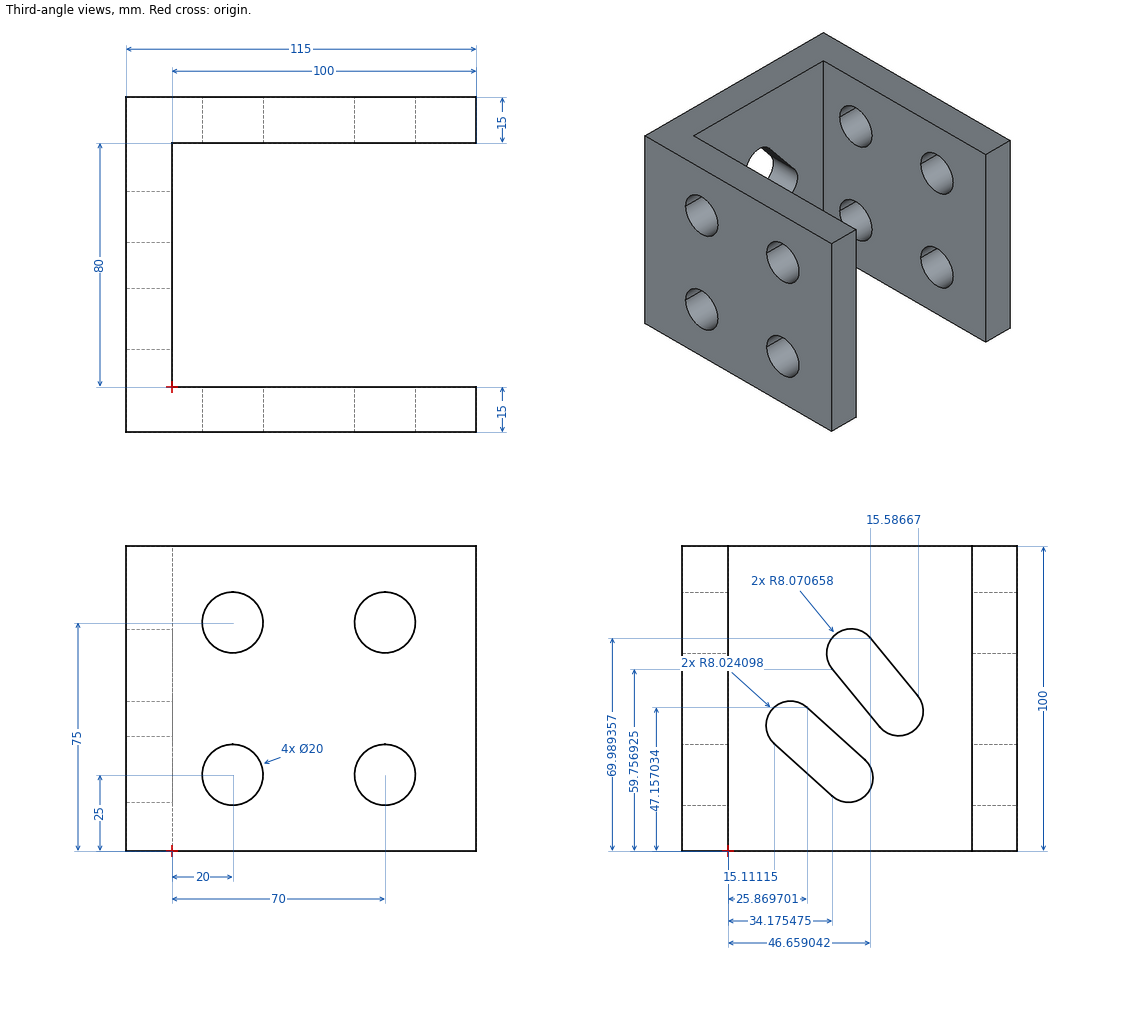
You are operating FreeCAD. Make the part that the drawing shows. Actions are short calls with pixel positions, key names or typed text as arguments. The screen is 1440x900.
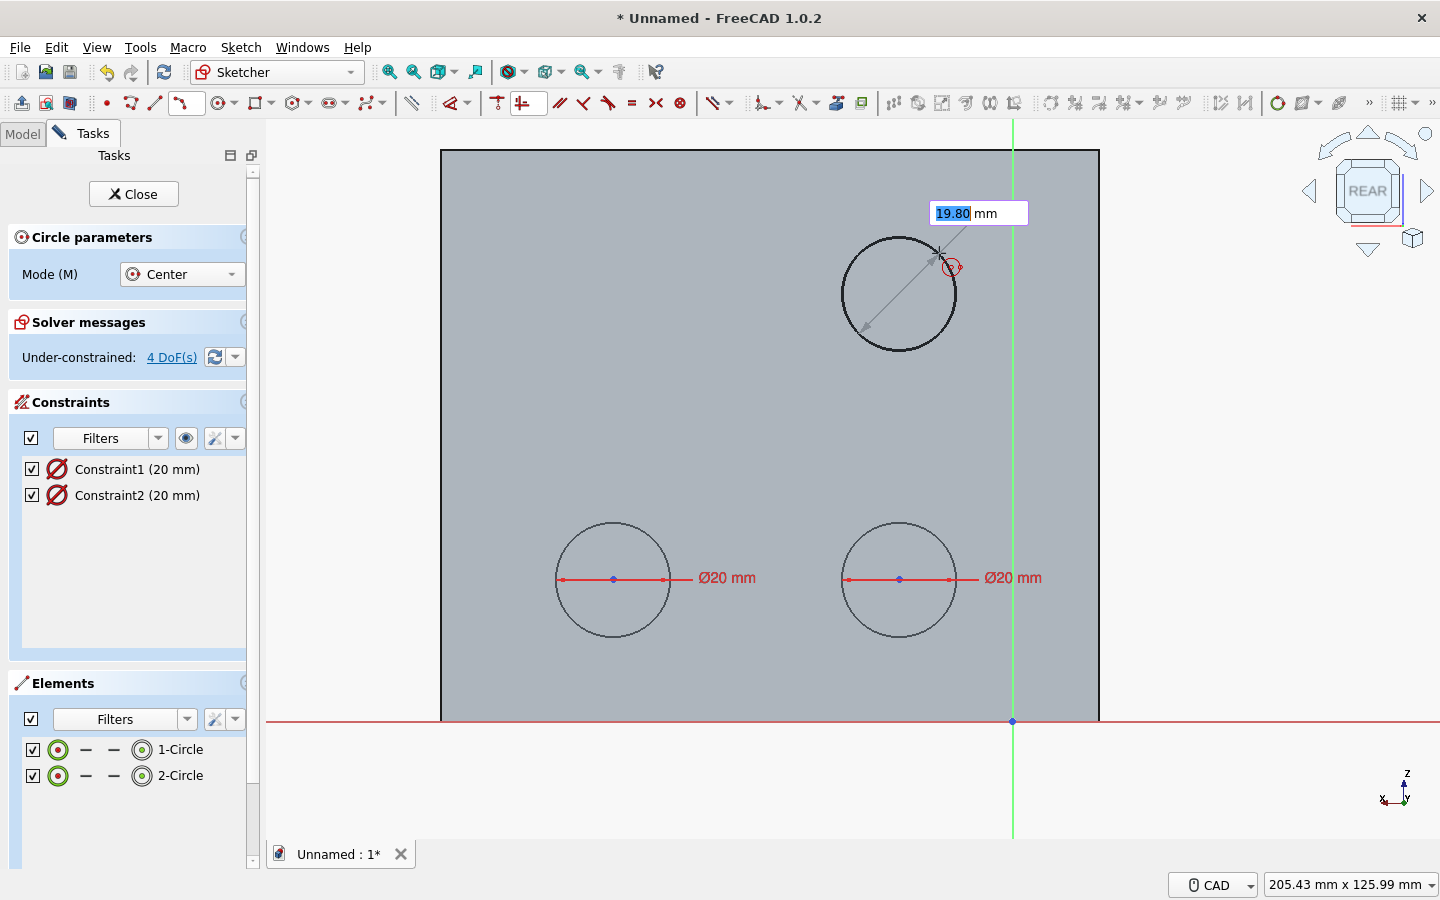
text(20)
key(Return)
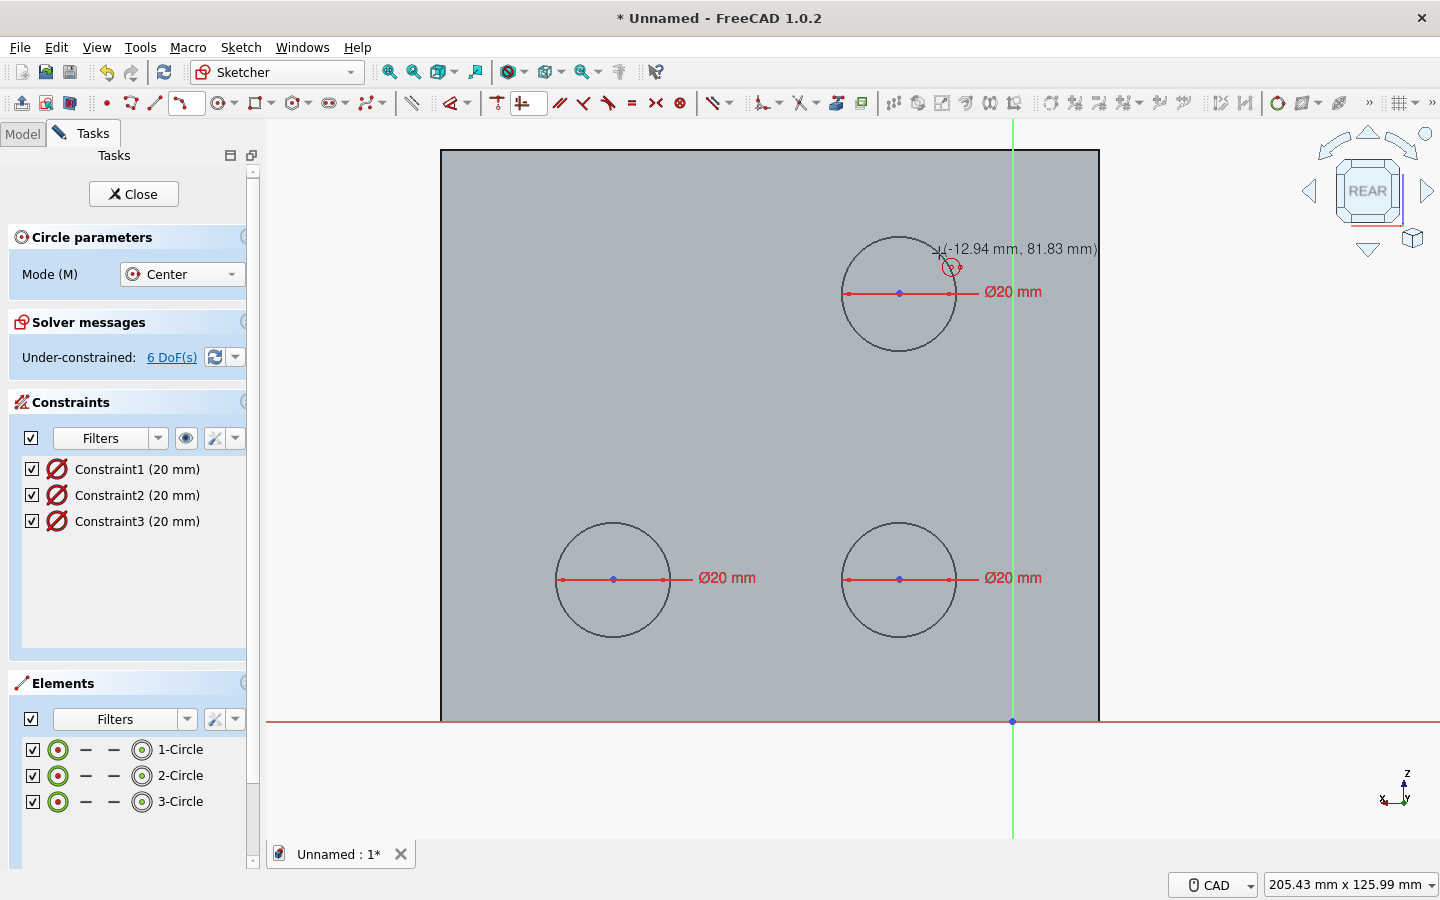
click(613, 293)
move(653, 253)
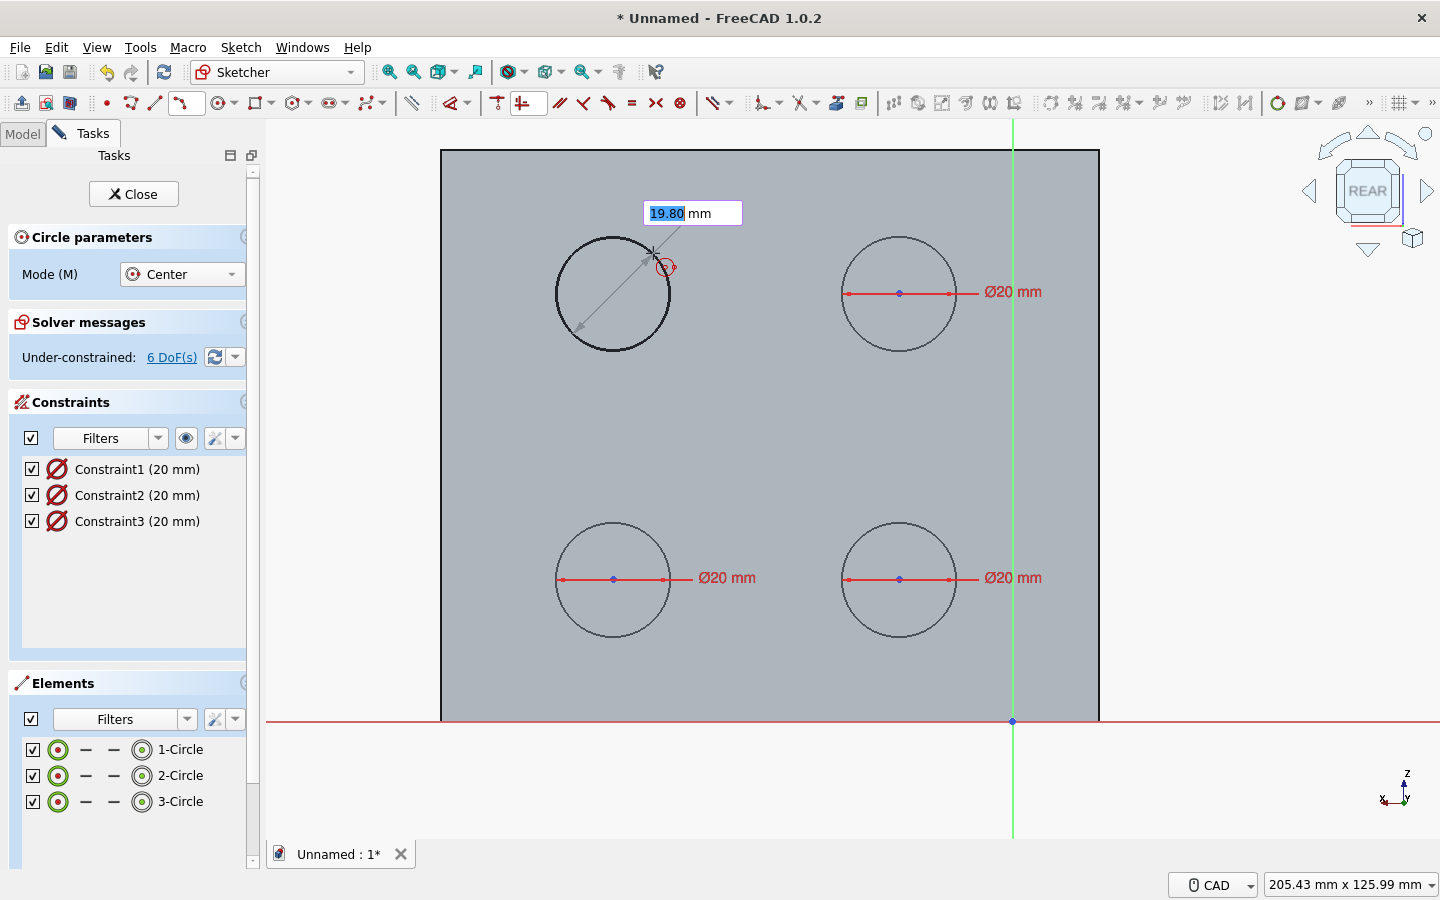
text(20)
key(Return)
key(Escape)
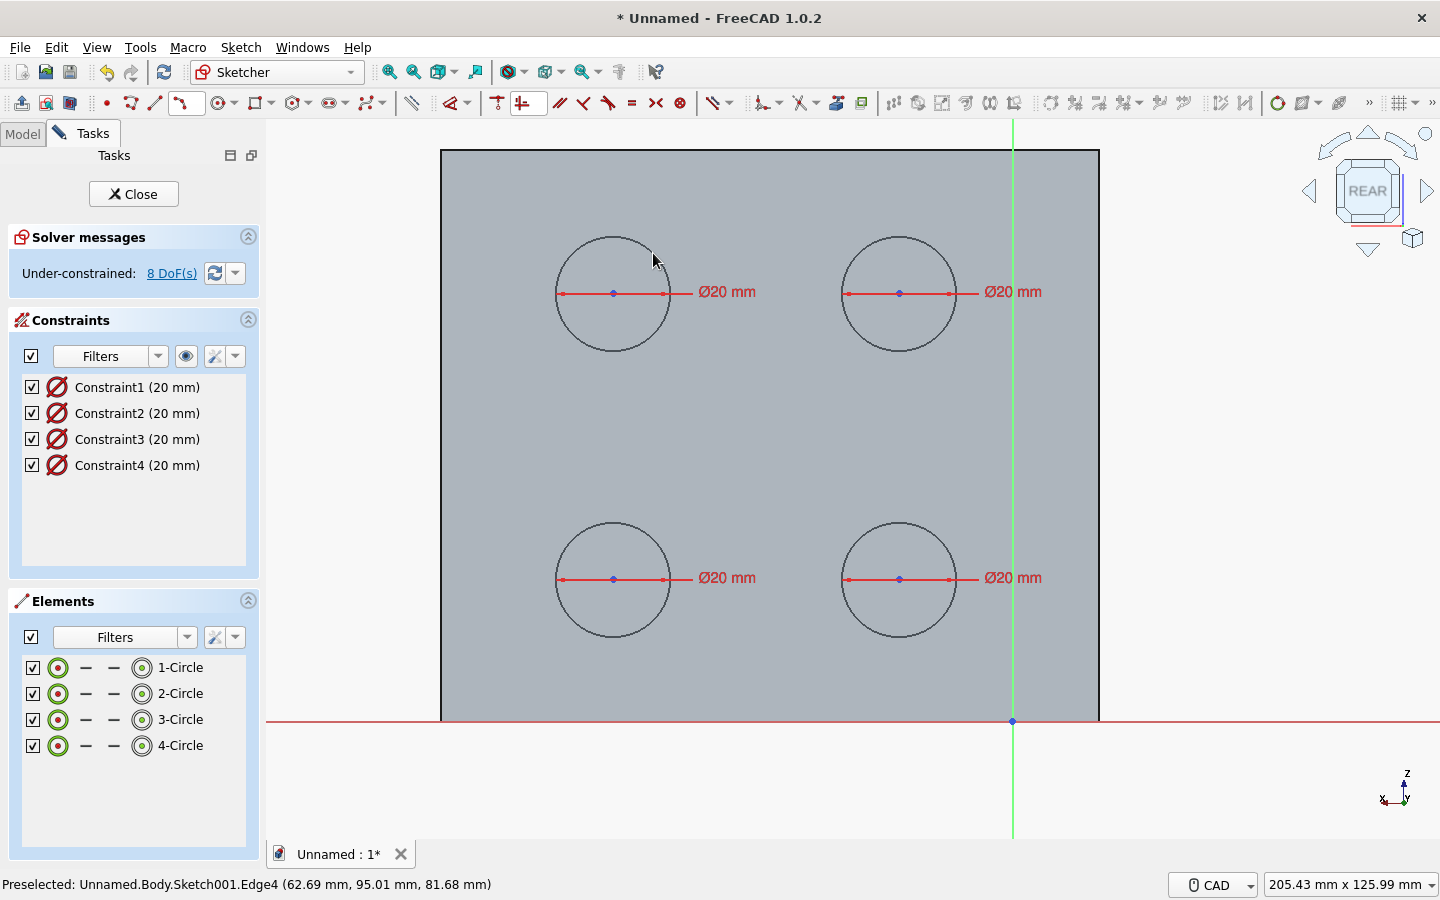
click(899, 580)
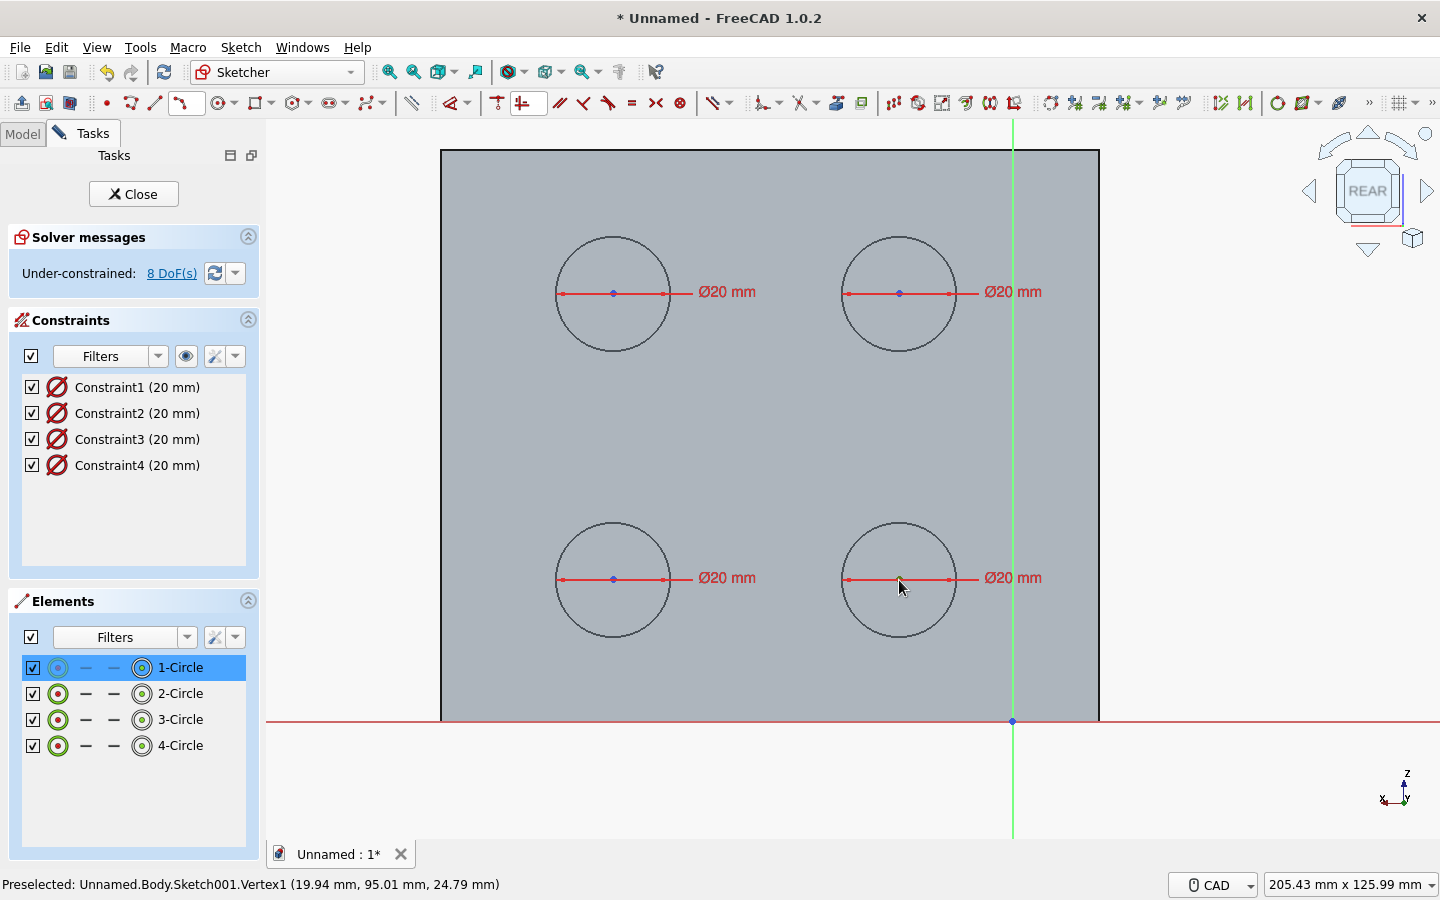
click(613, 580)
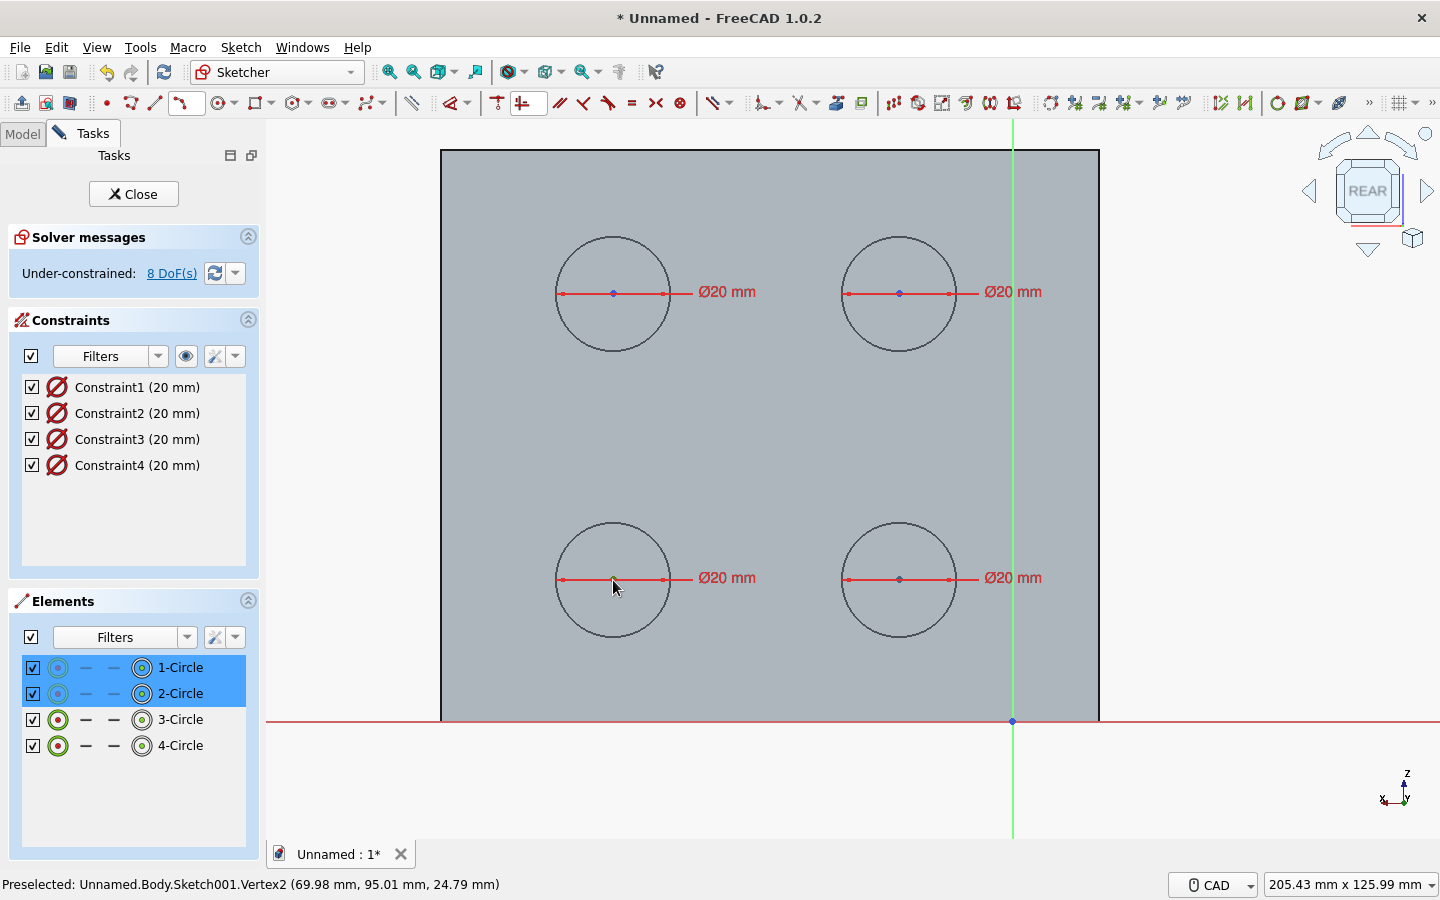
key(h)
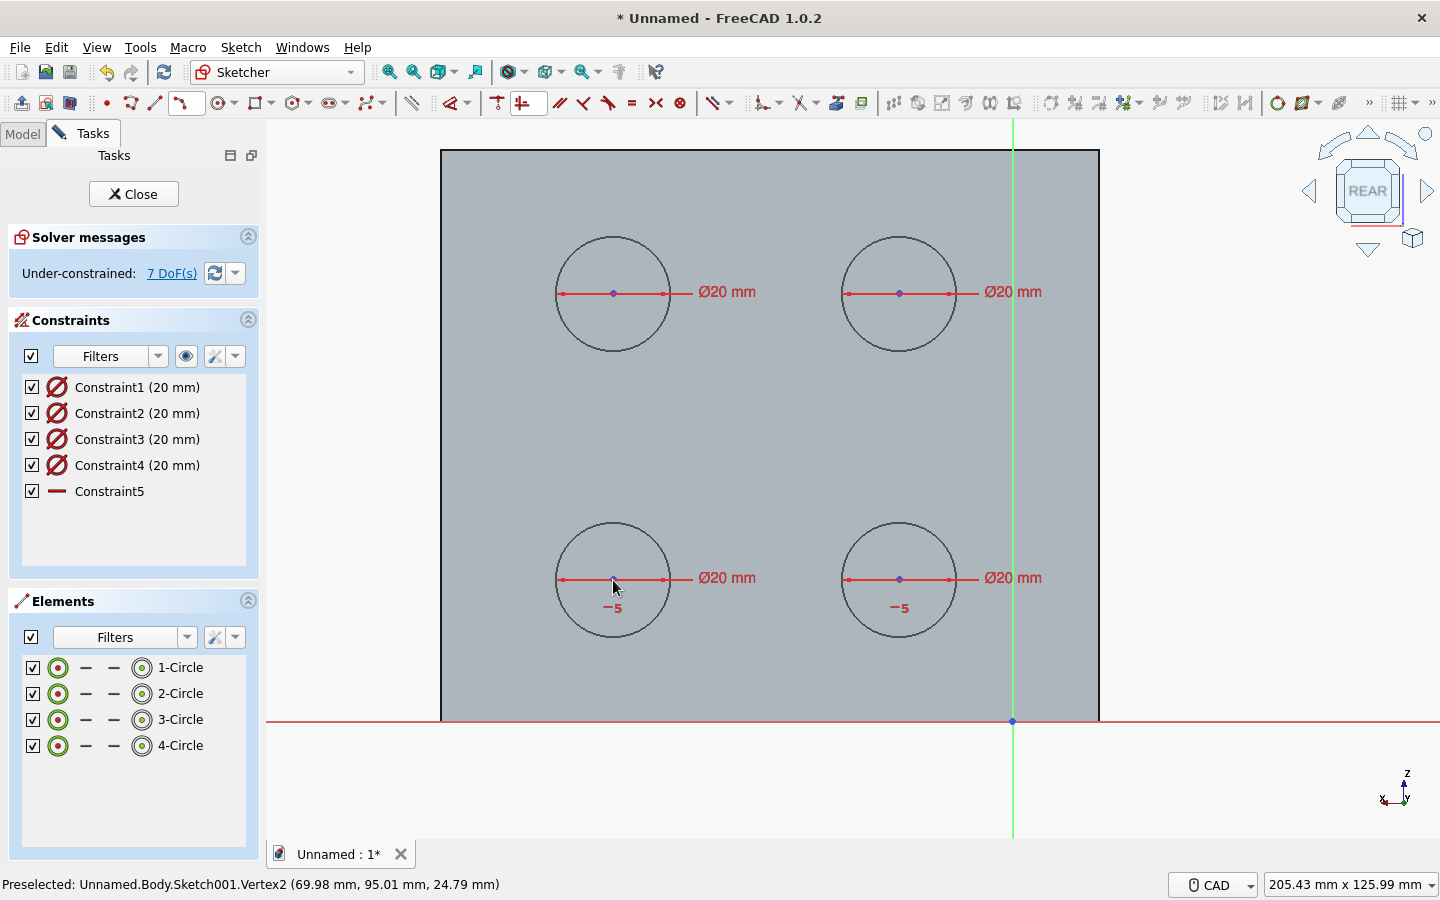
click(899, 580)